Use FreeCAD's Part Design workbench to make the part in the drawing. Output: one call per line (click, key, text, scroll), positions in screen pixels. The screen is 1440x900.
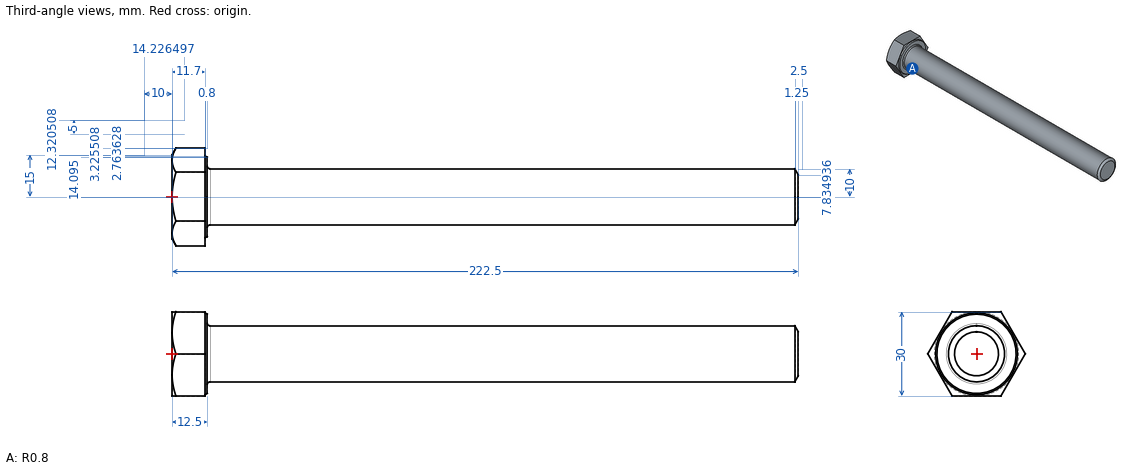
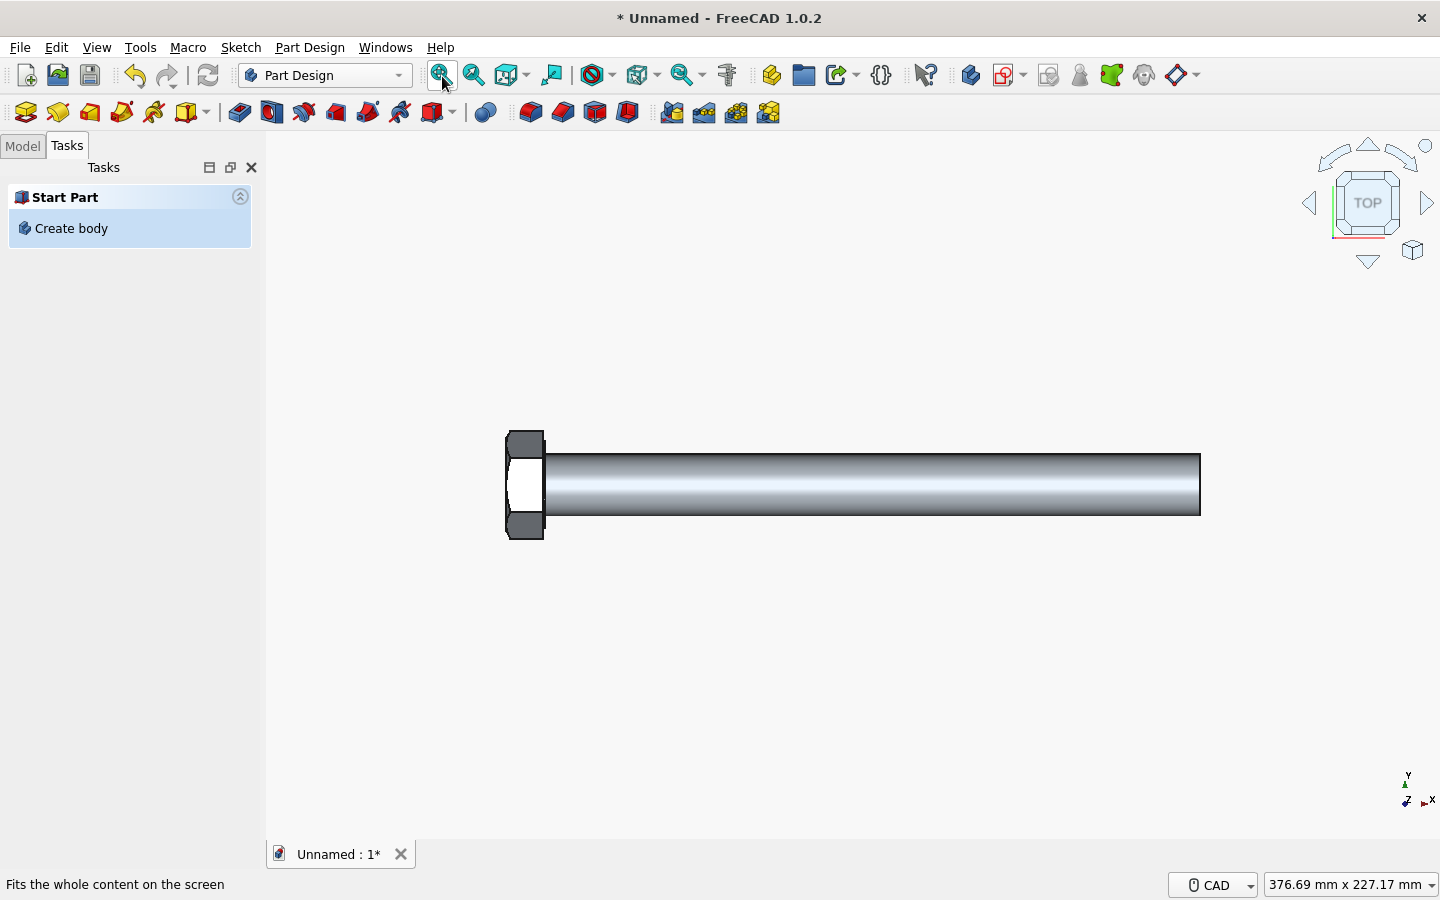
key(1)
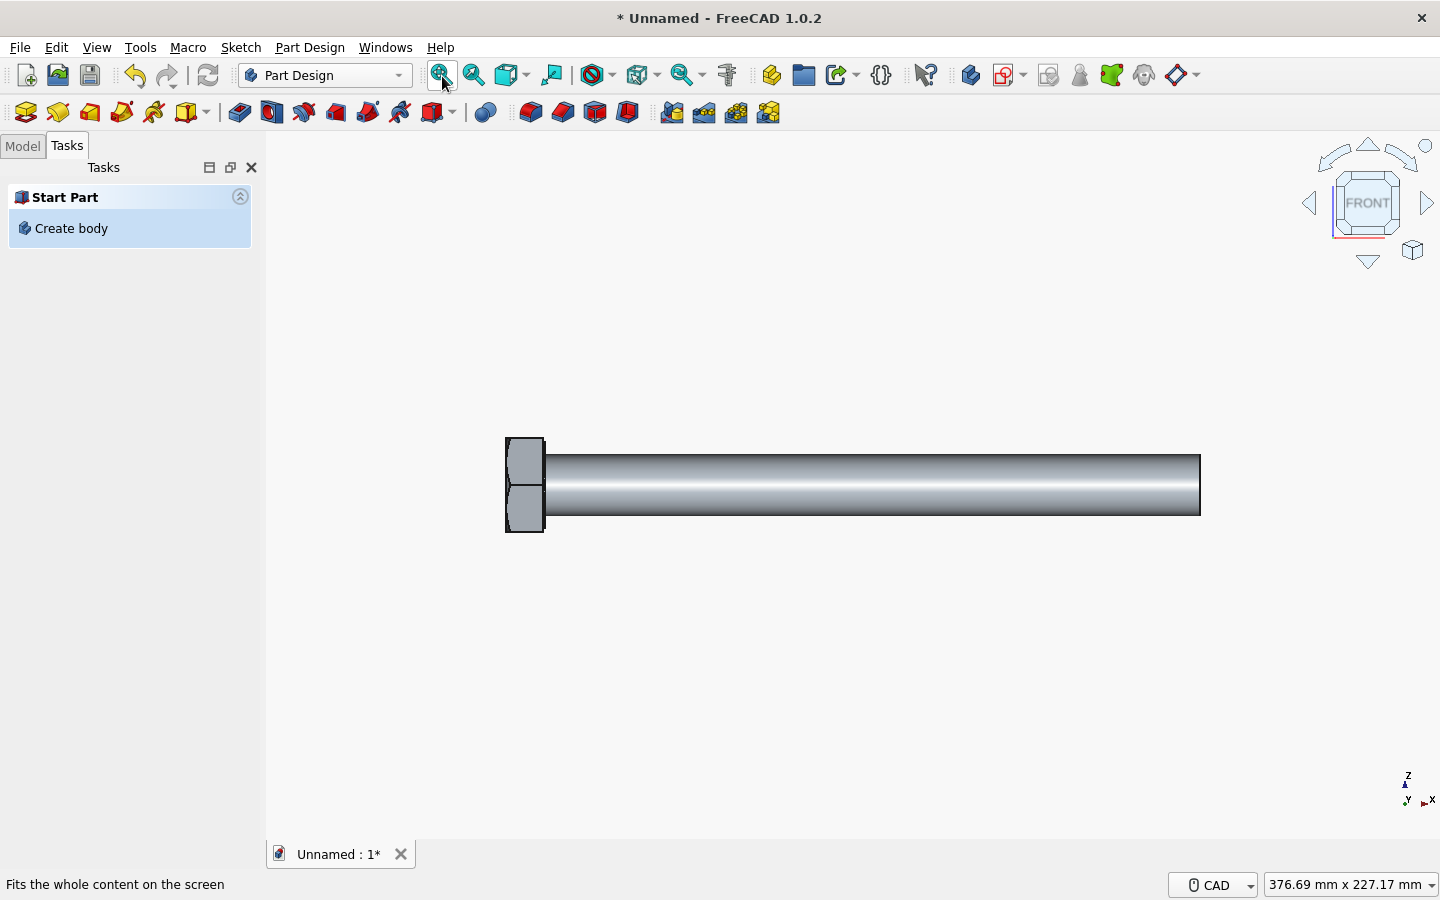
key(3)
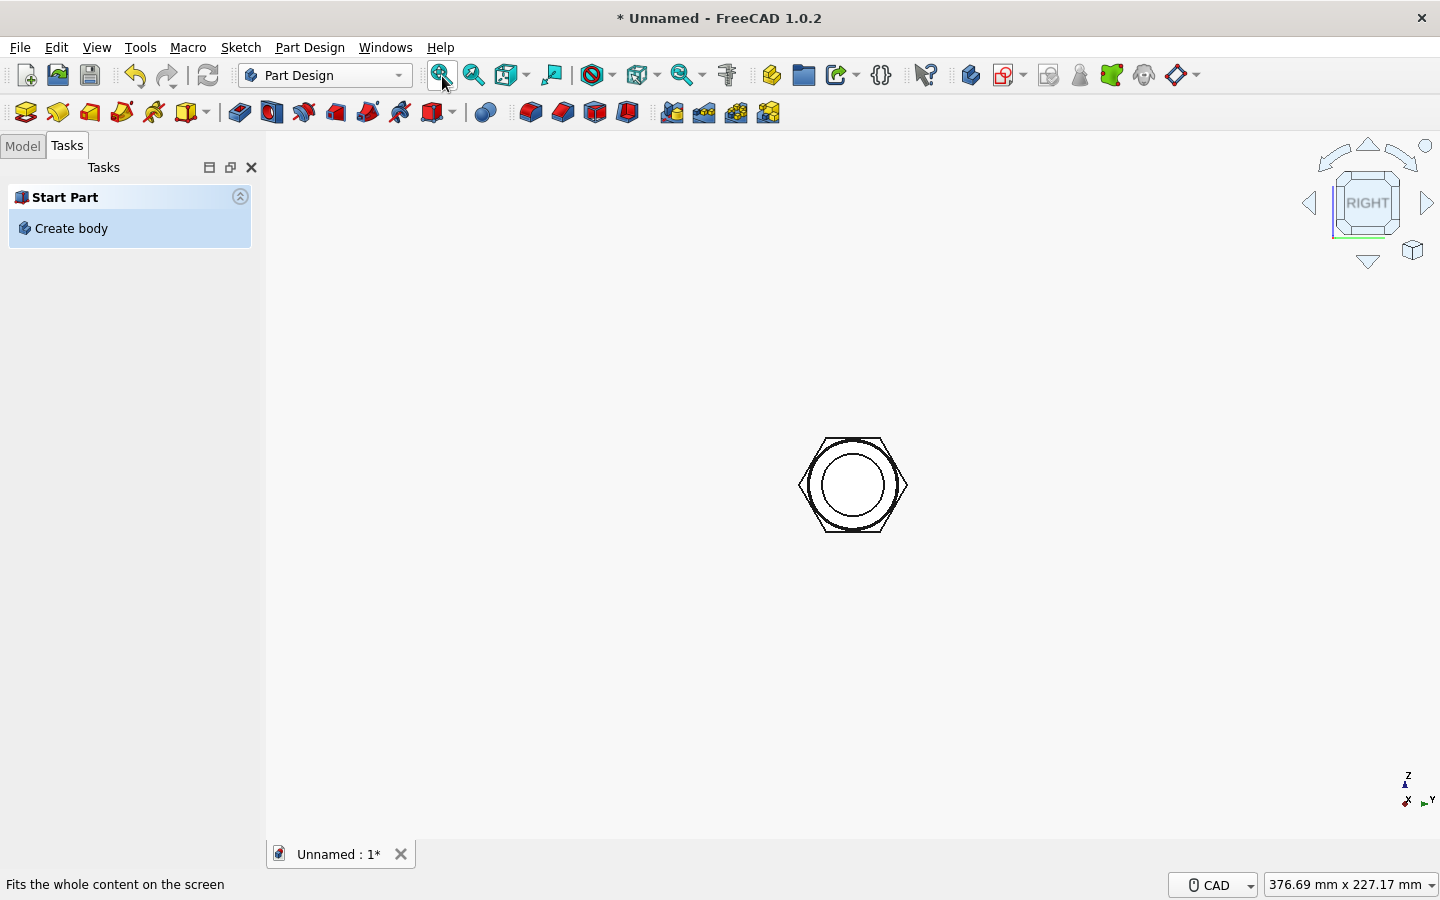
click(442, 76)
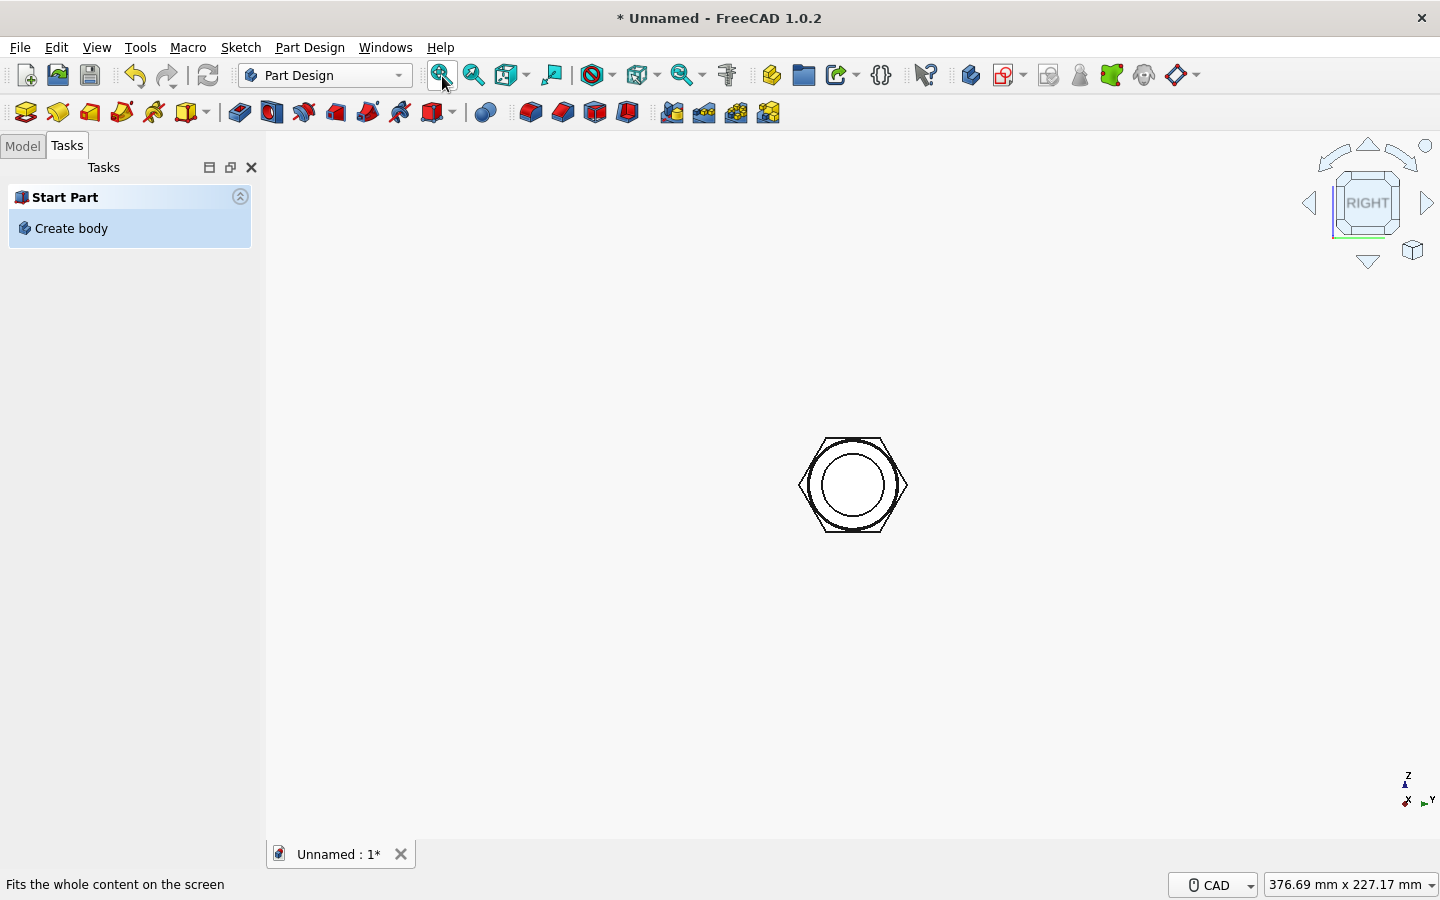
key(5)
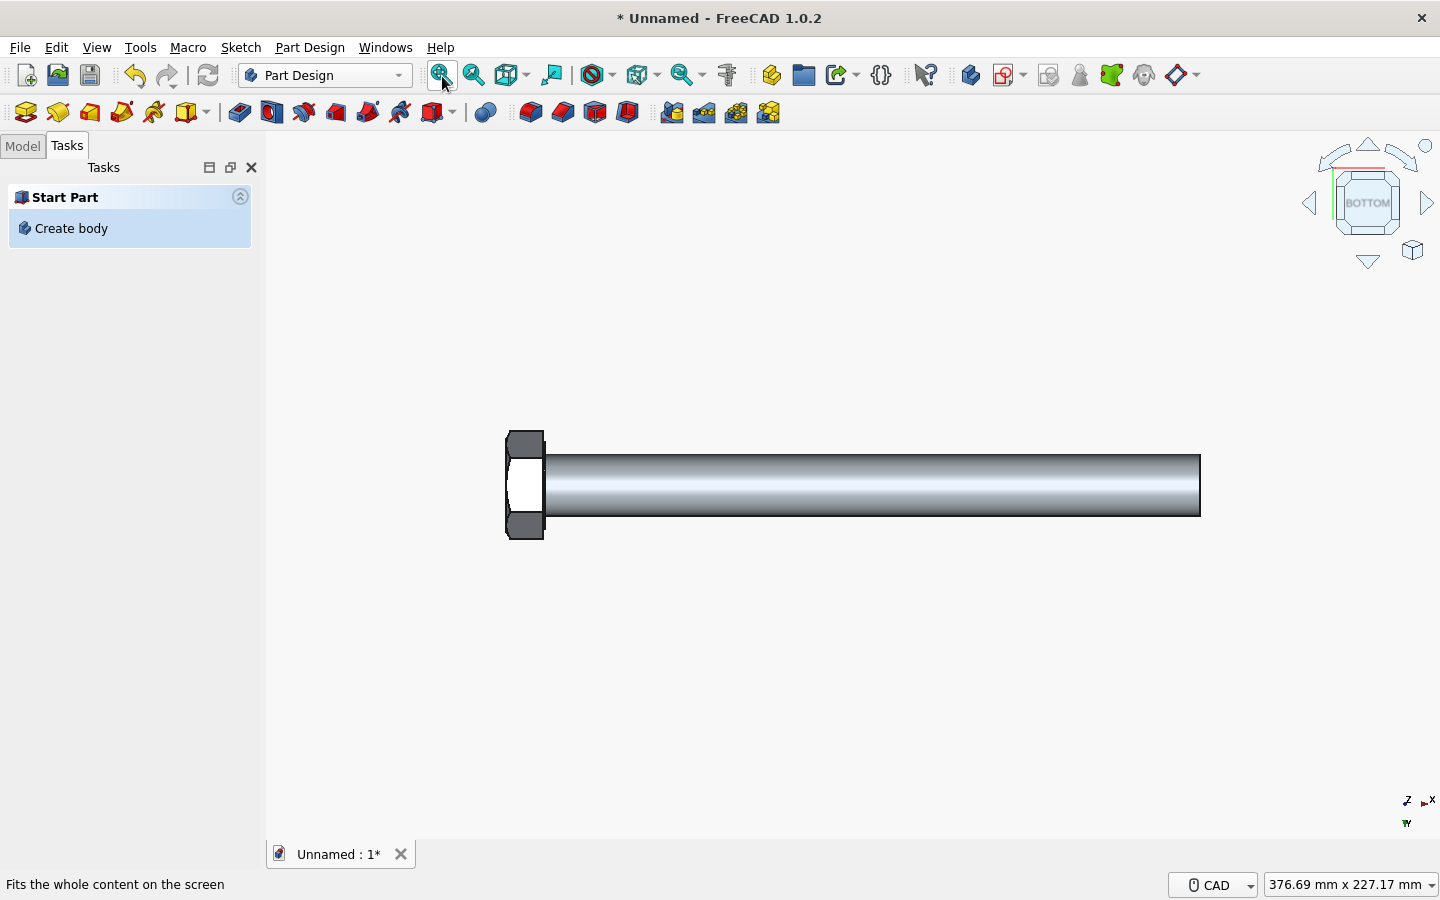
key(4)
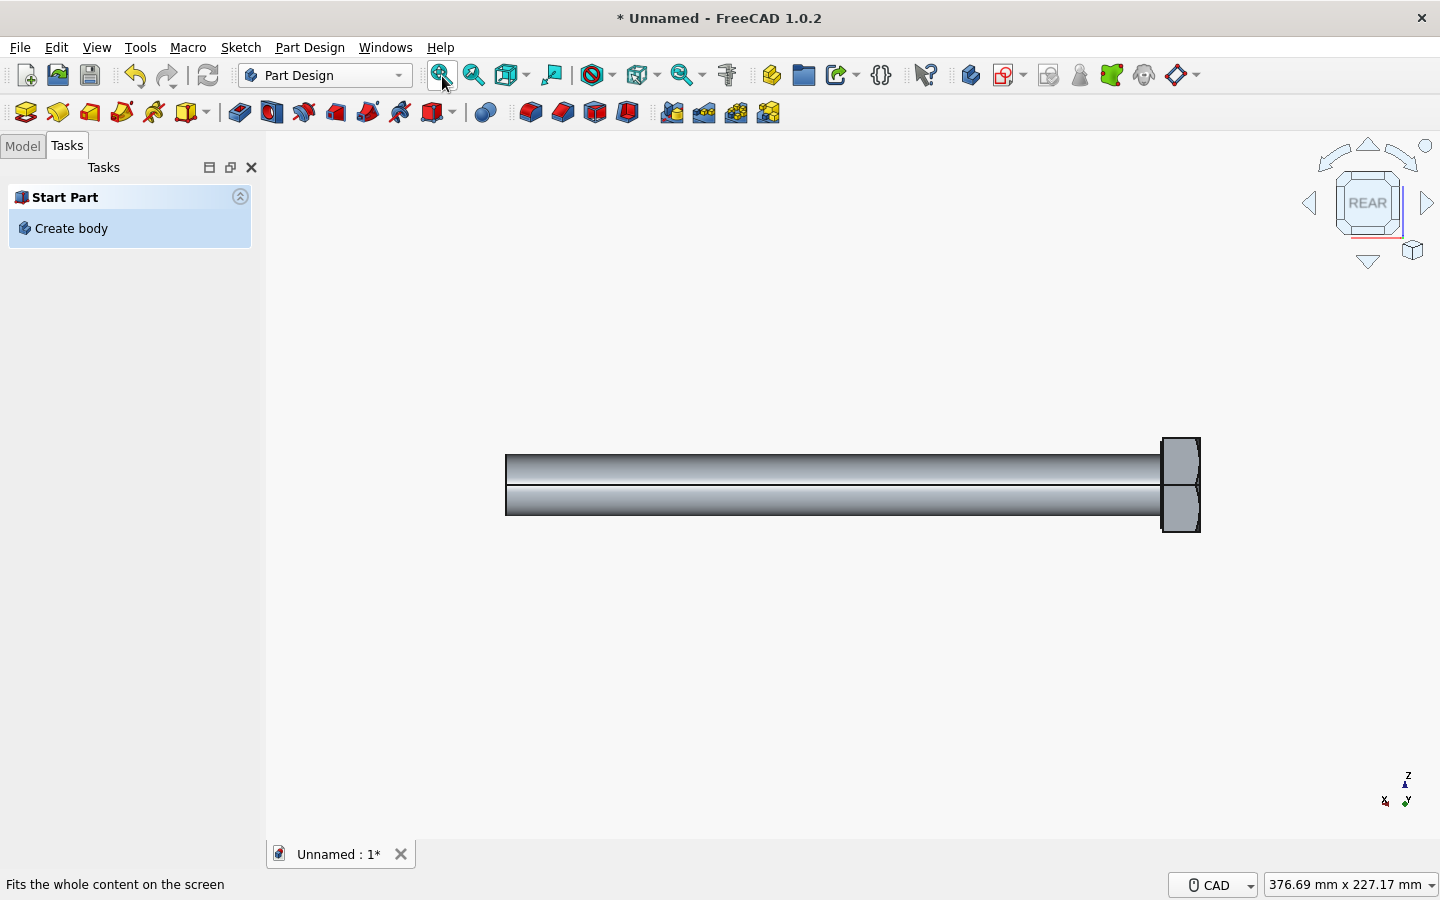
key(6)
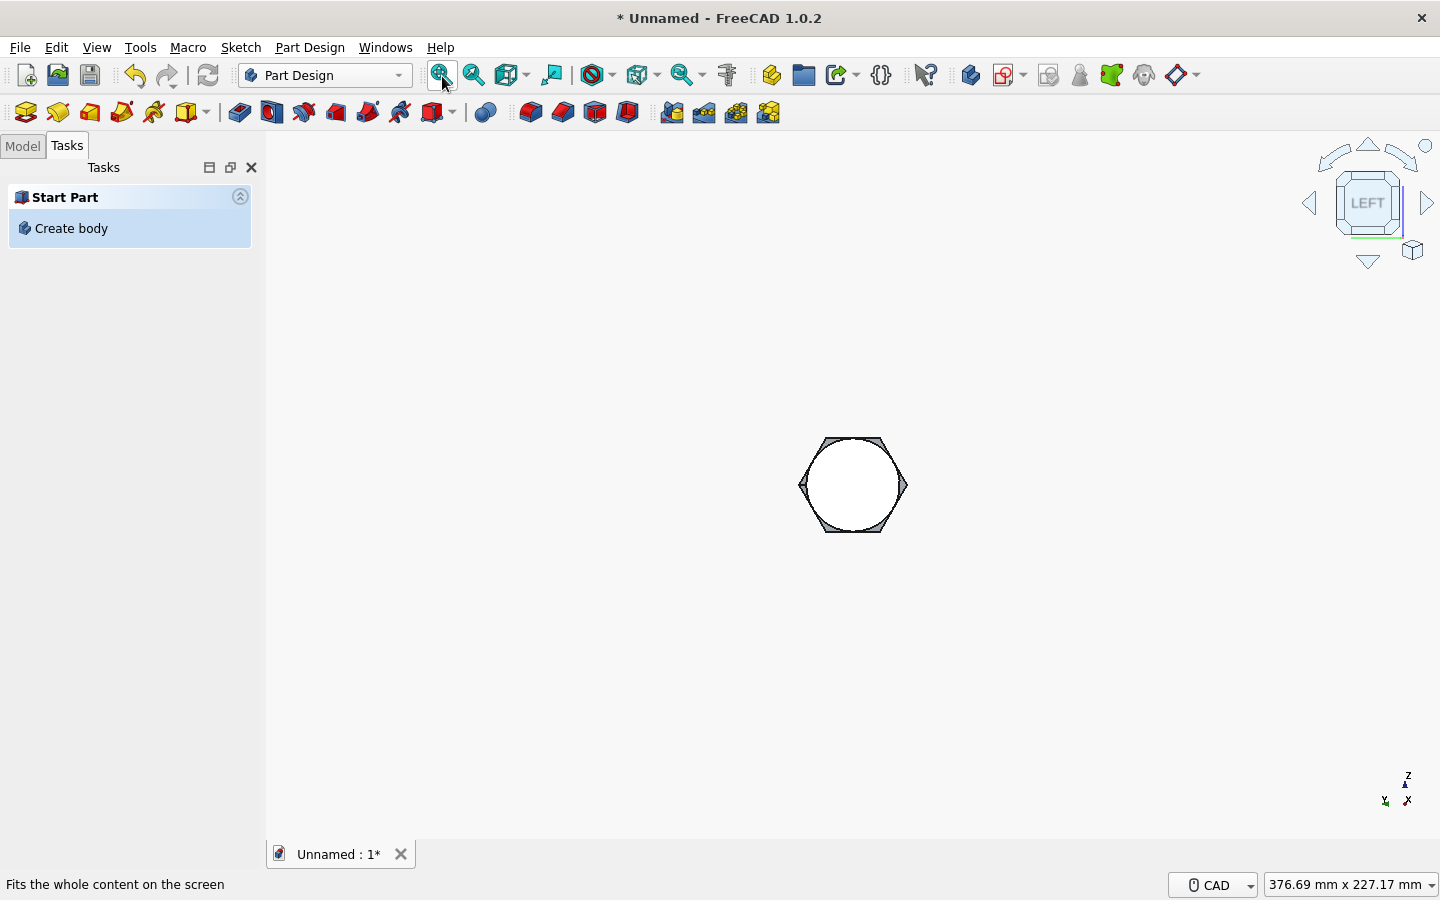
click(442, 76)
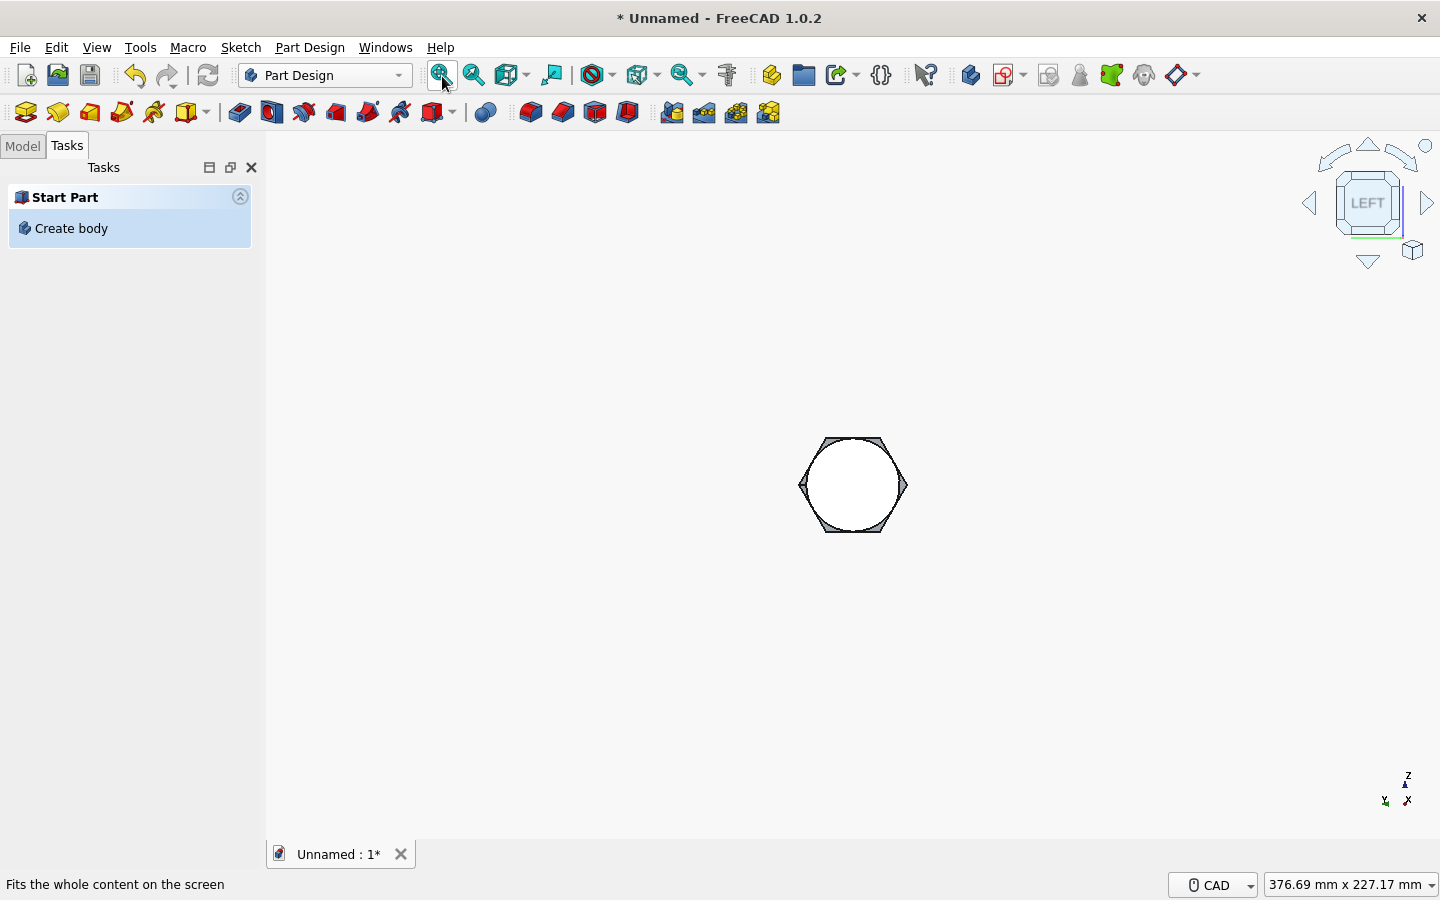
key(v)
key(3)